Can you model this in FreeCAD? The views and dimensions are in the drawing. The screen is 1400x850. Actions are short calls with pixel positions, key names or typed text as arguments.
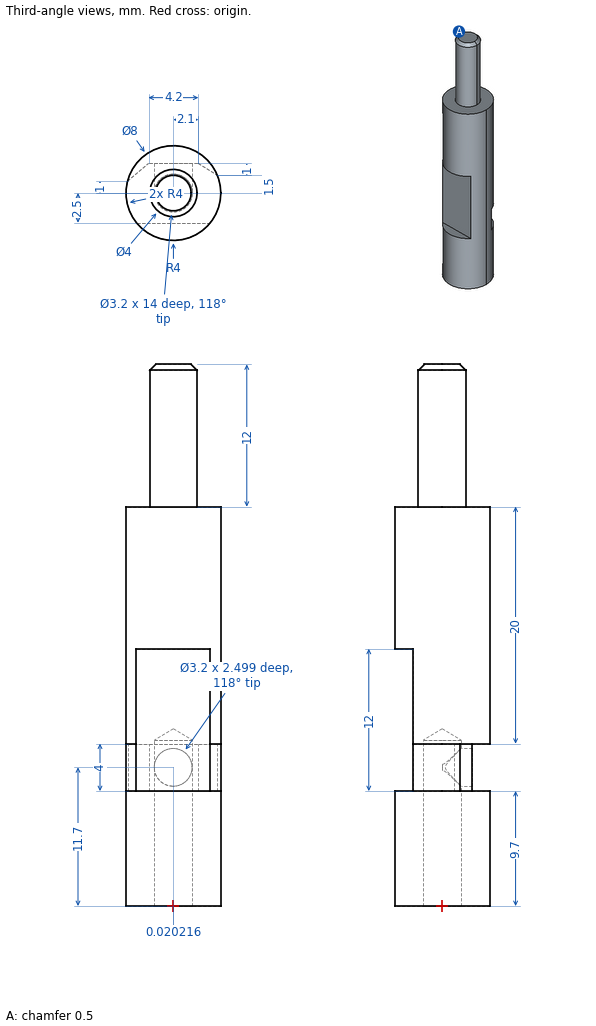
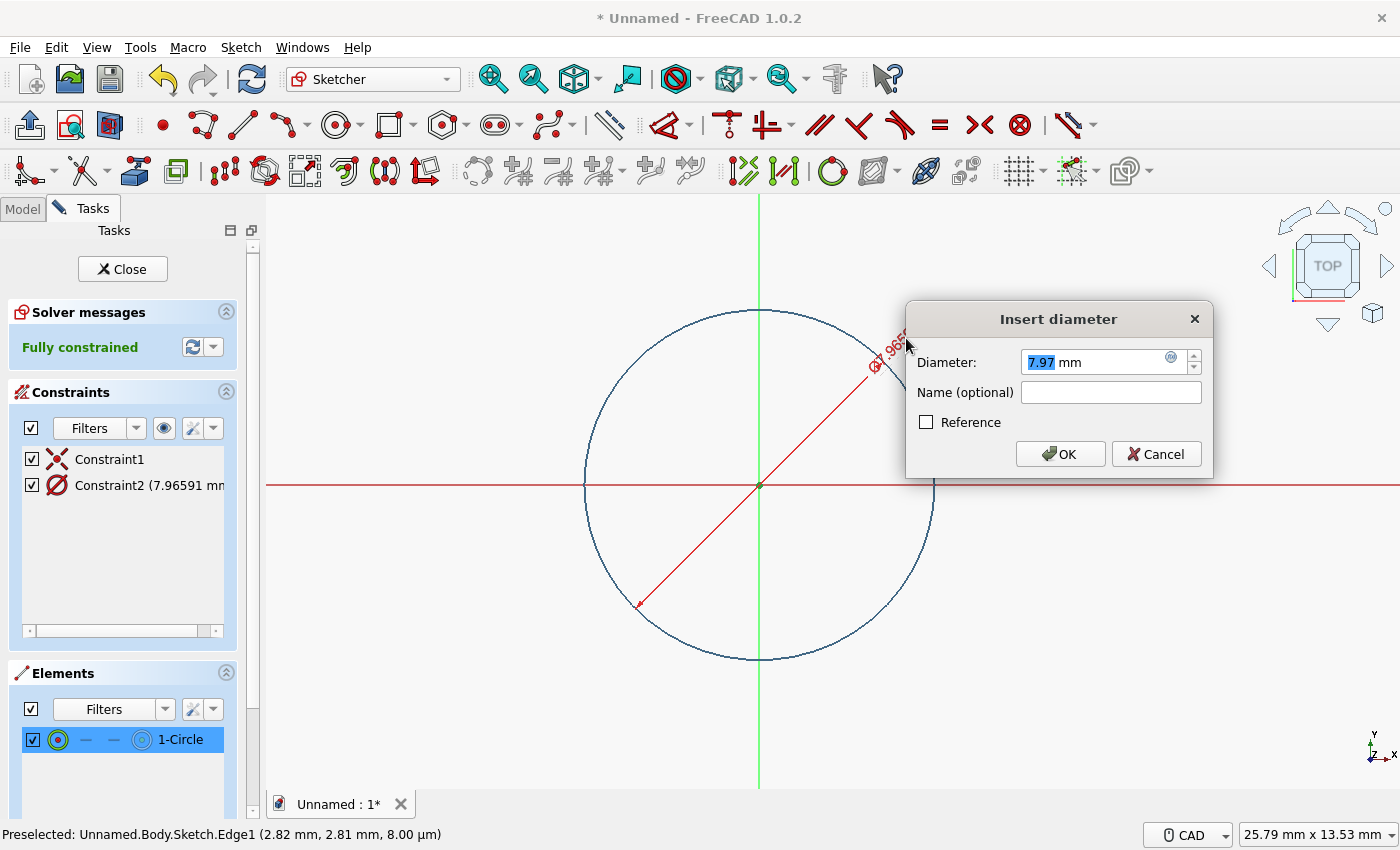
text(8)
key(Return)
key(Escape)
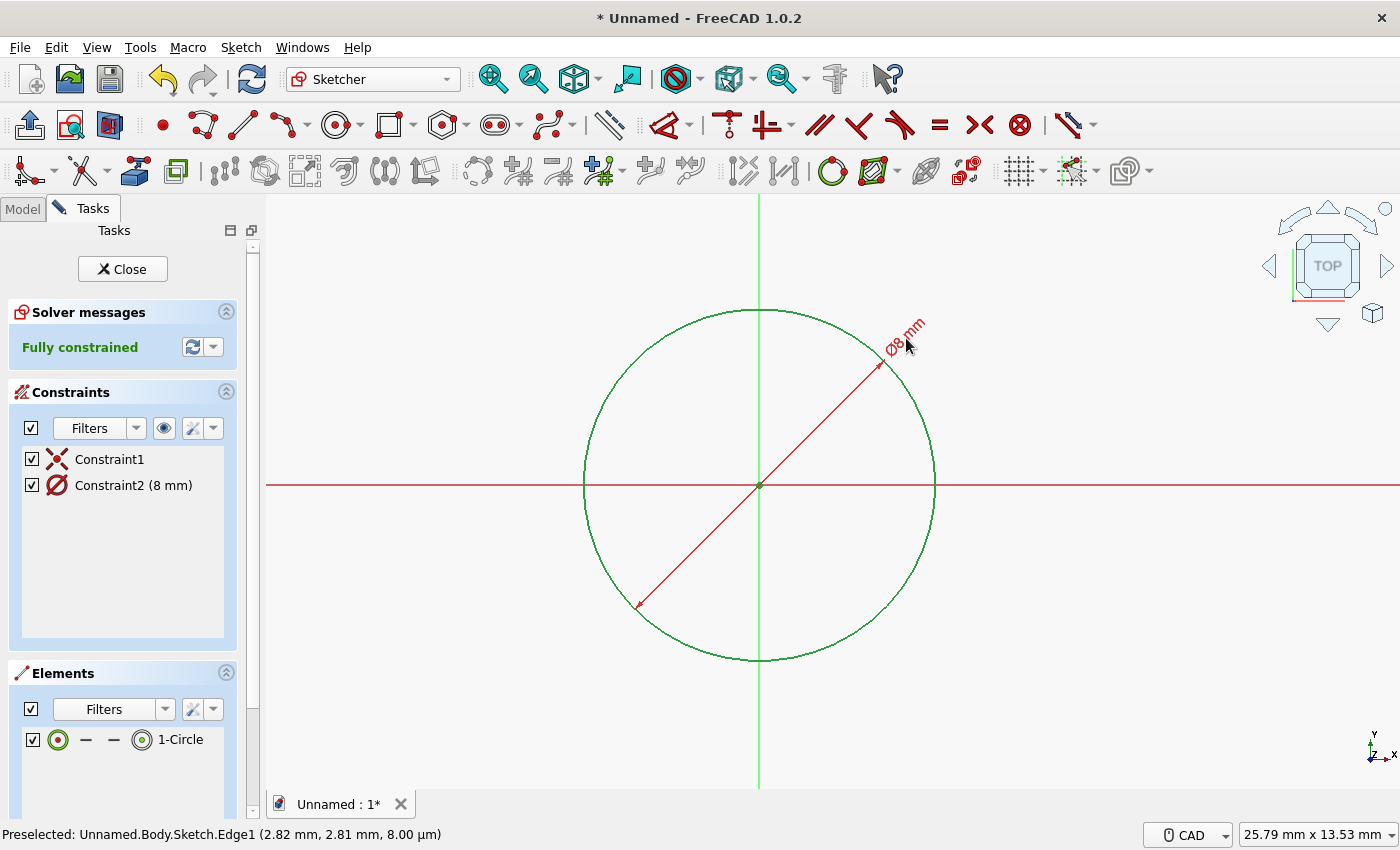
click(123, 269)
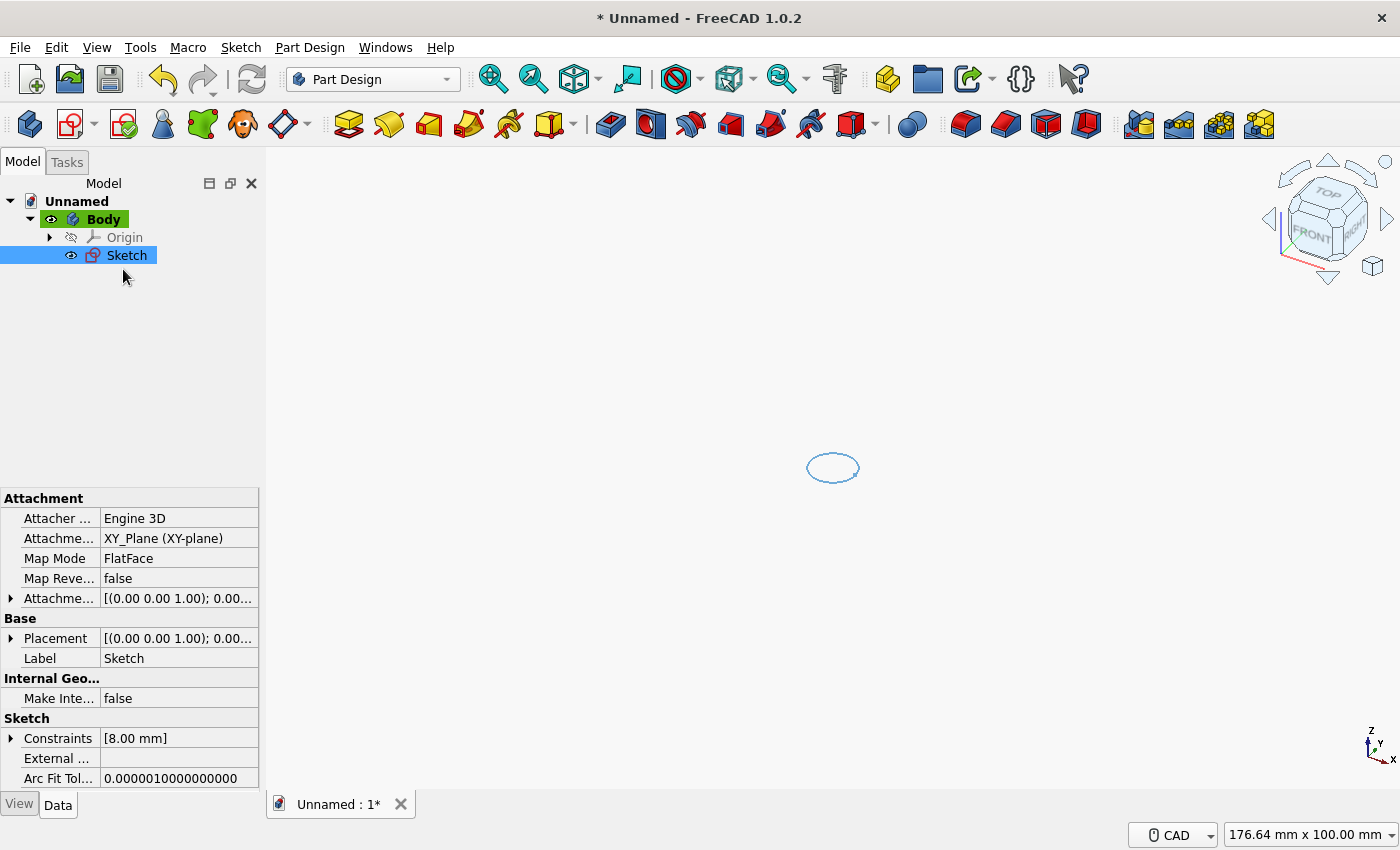
click(350, 124)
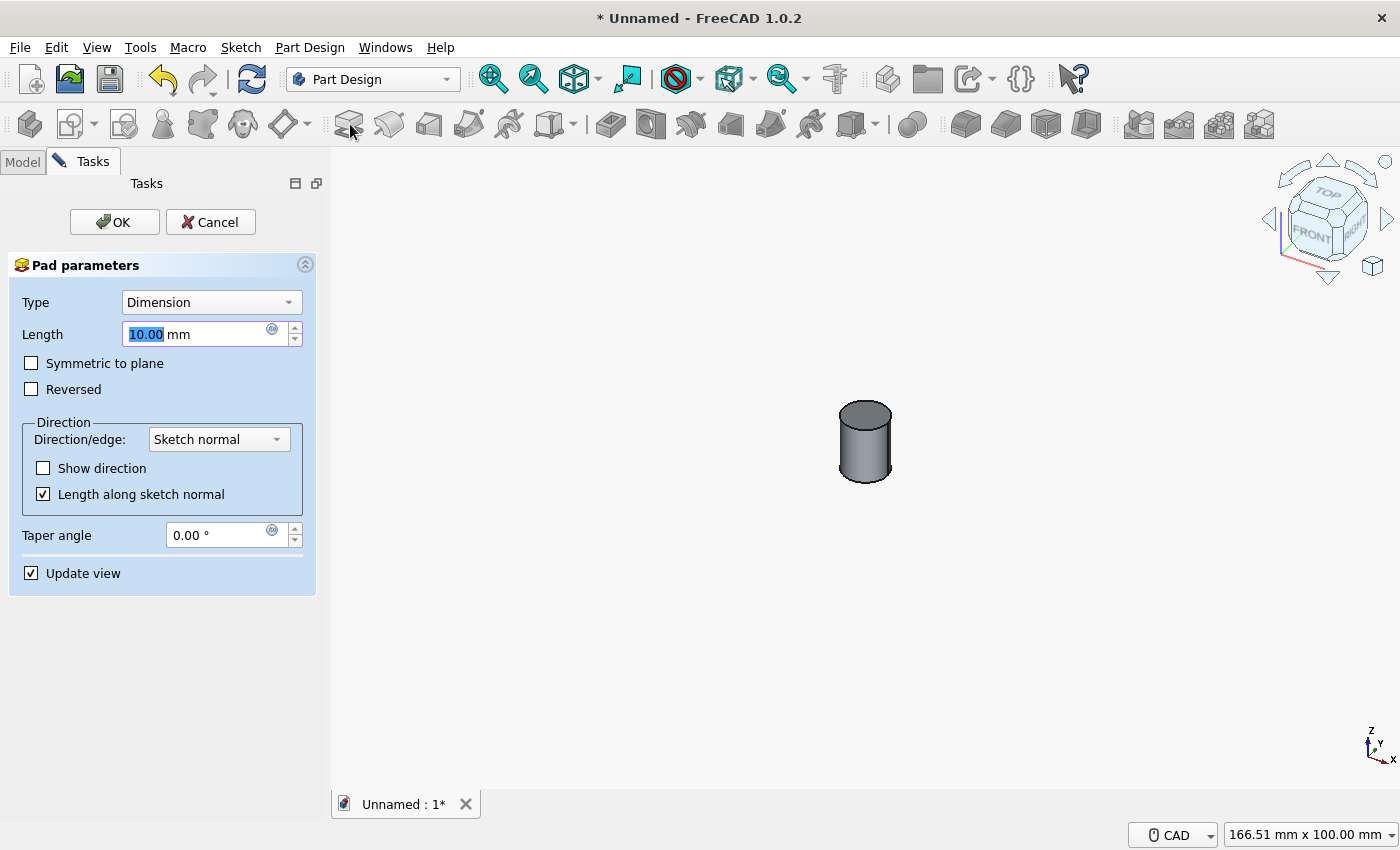
text(9.7)
key(Tab)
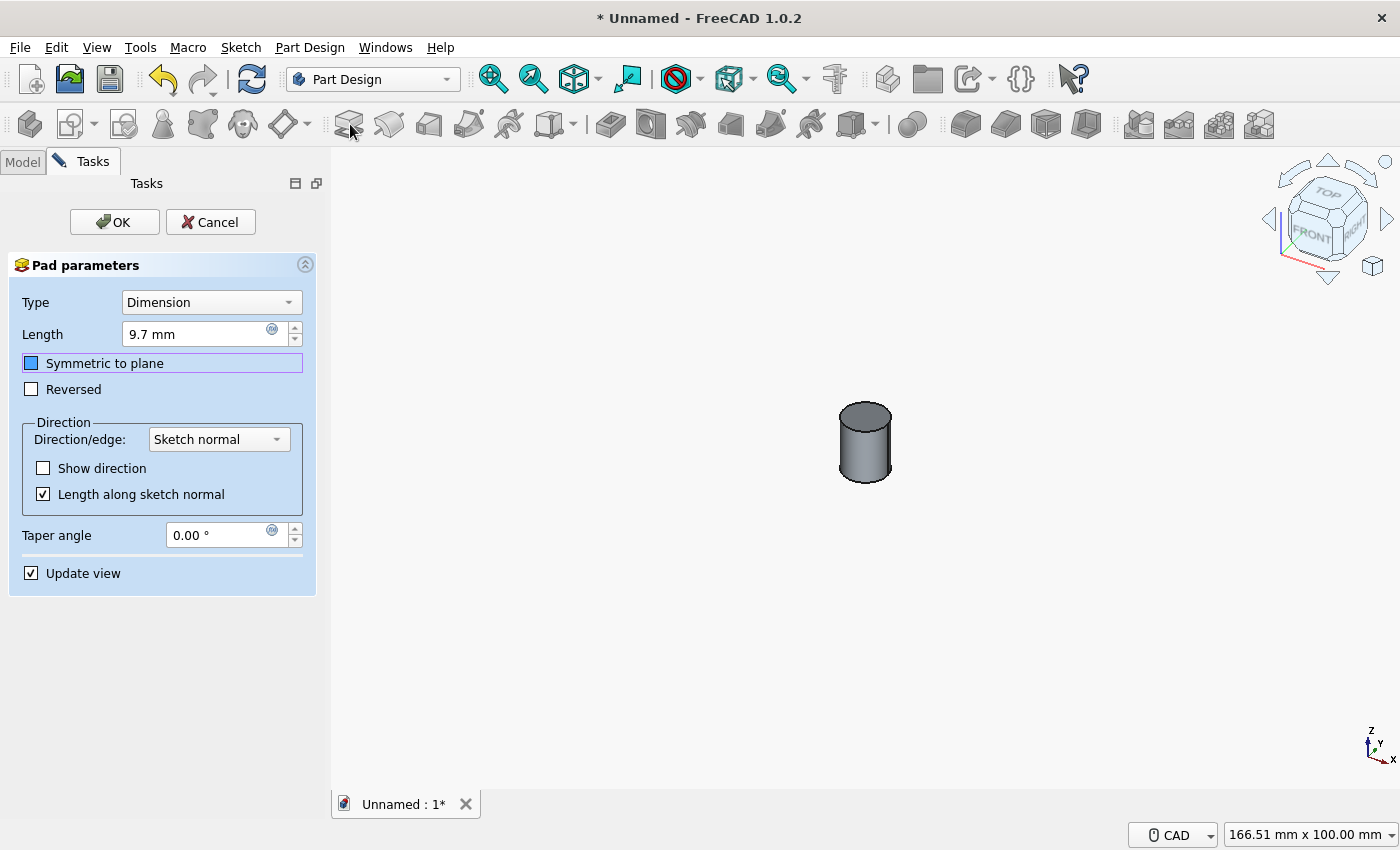
click(115, 222)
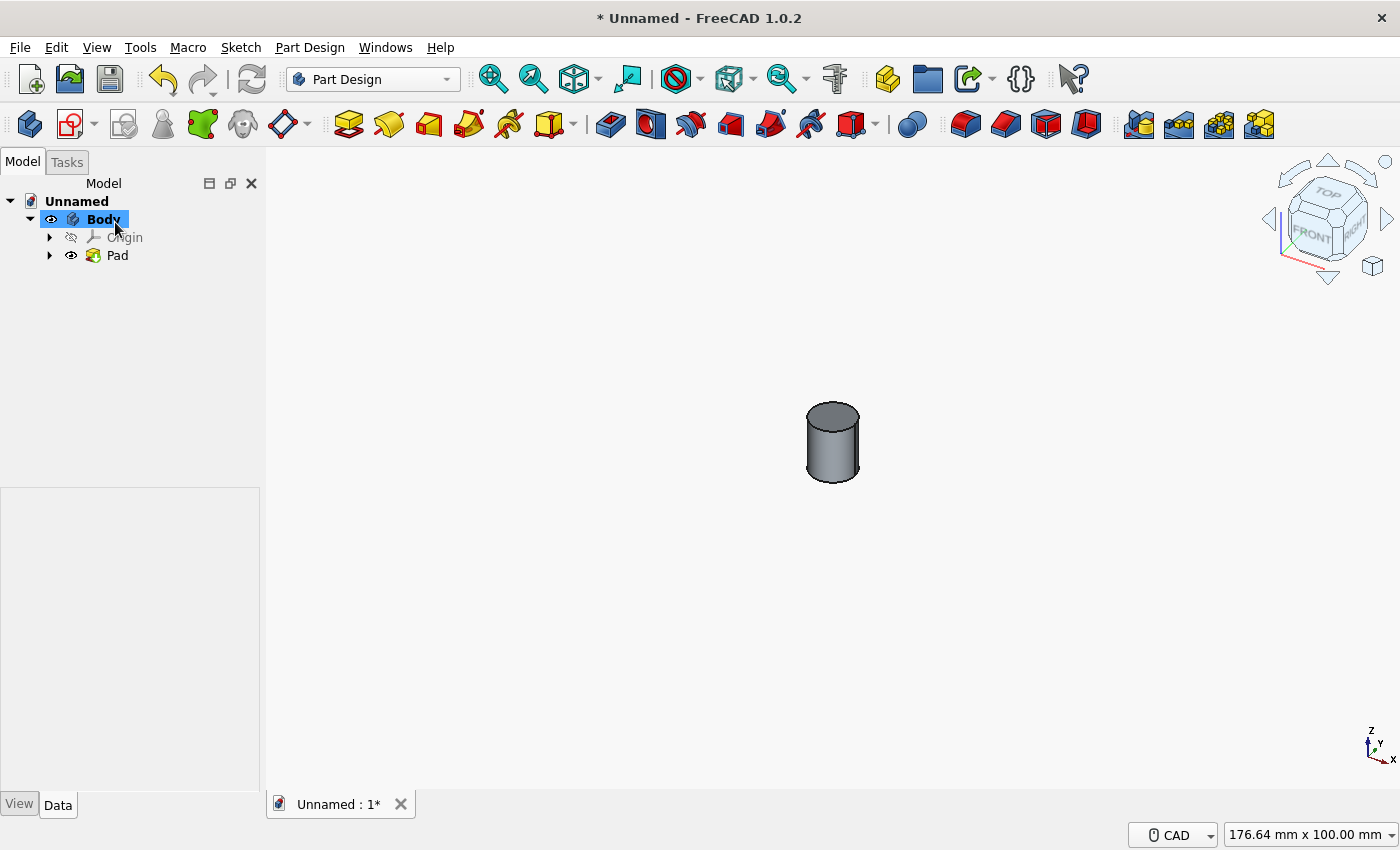
click(494, 80)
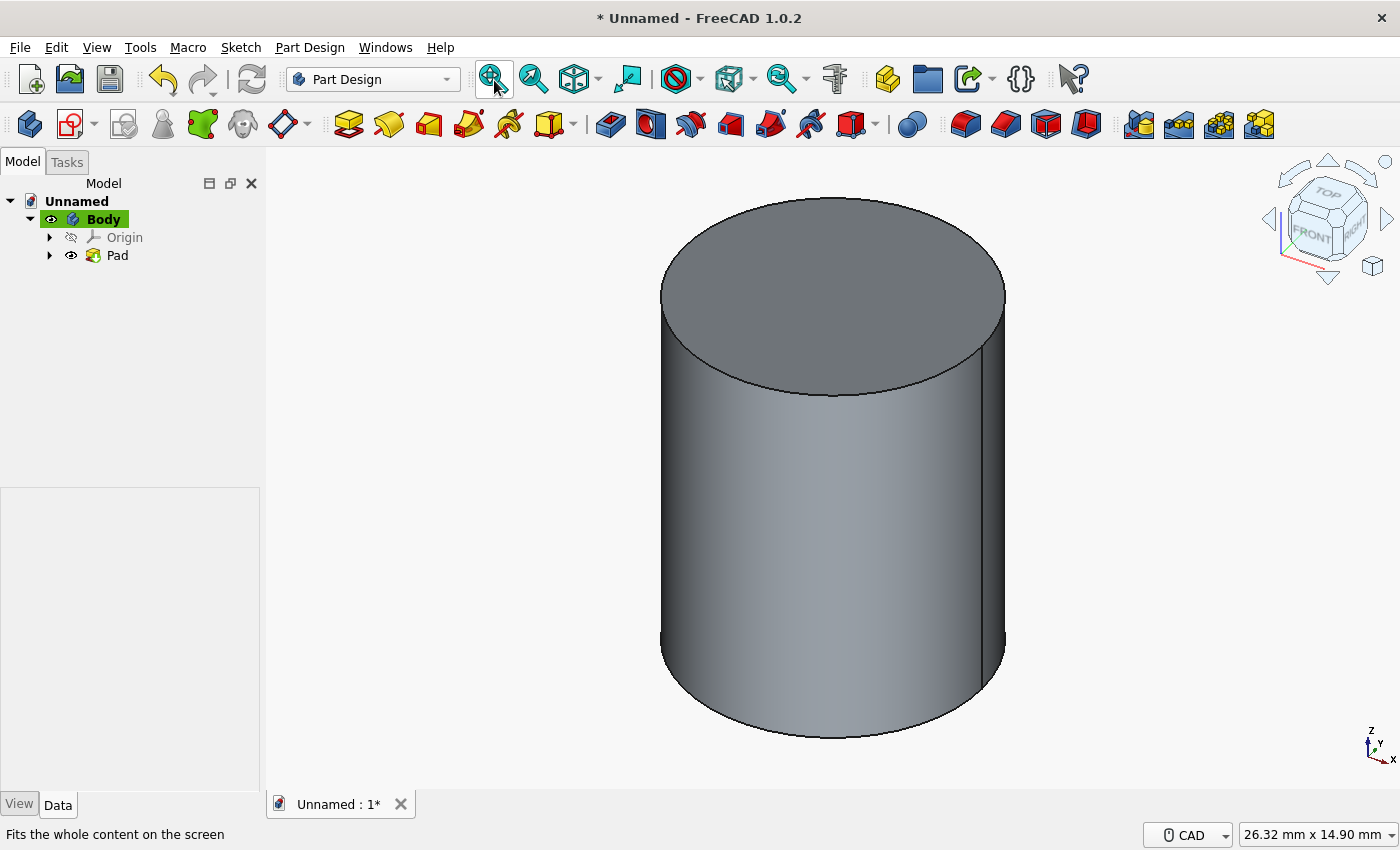
click(833, 296)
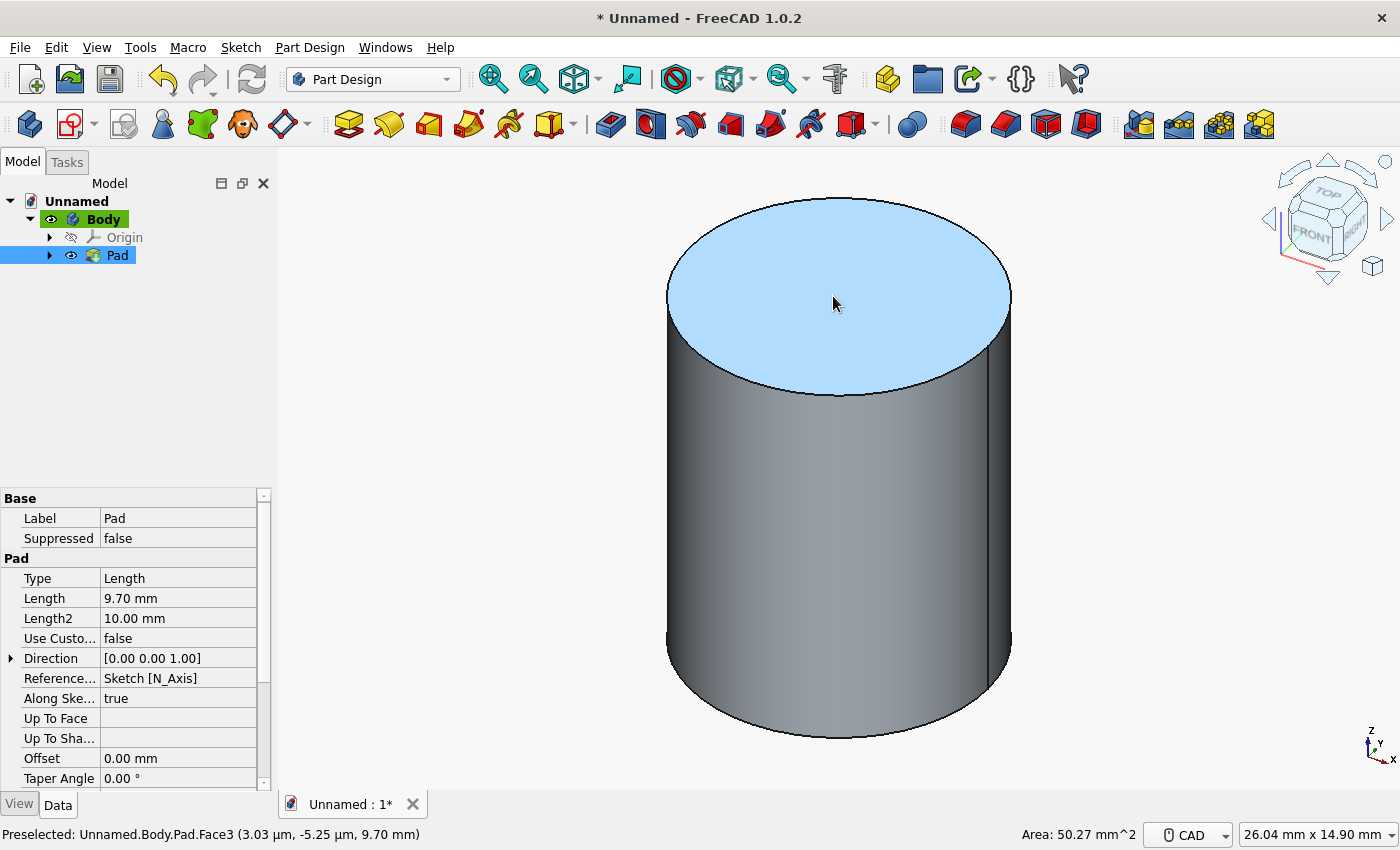
click(70, 124)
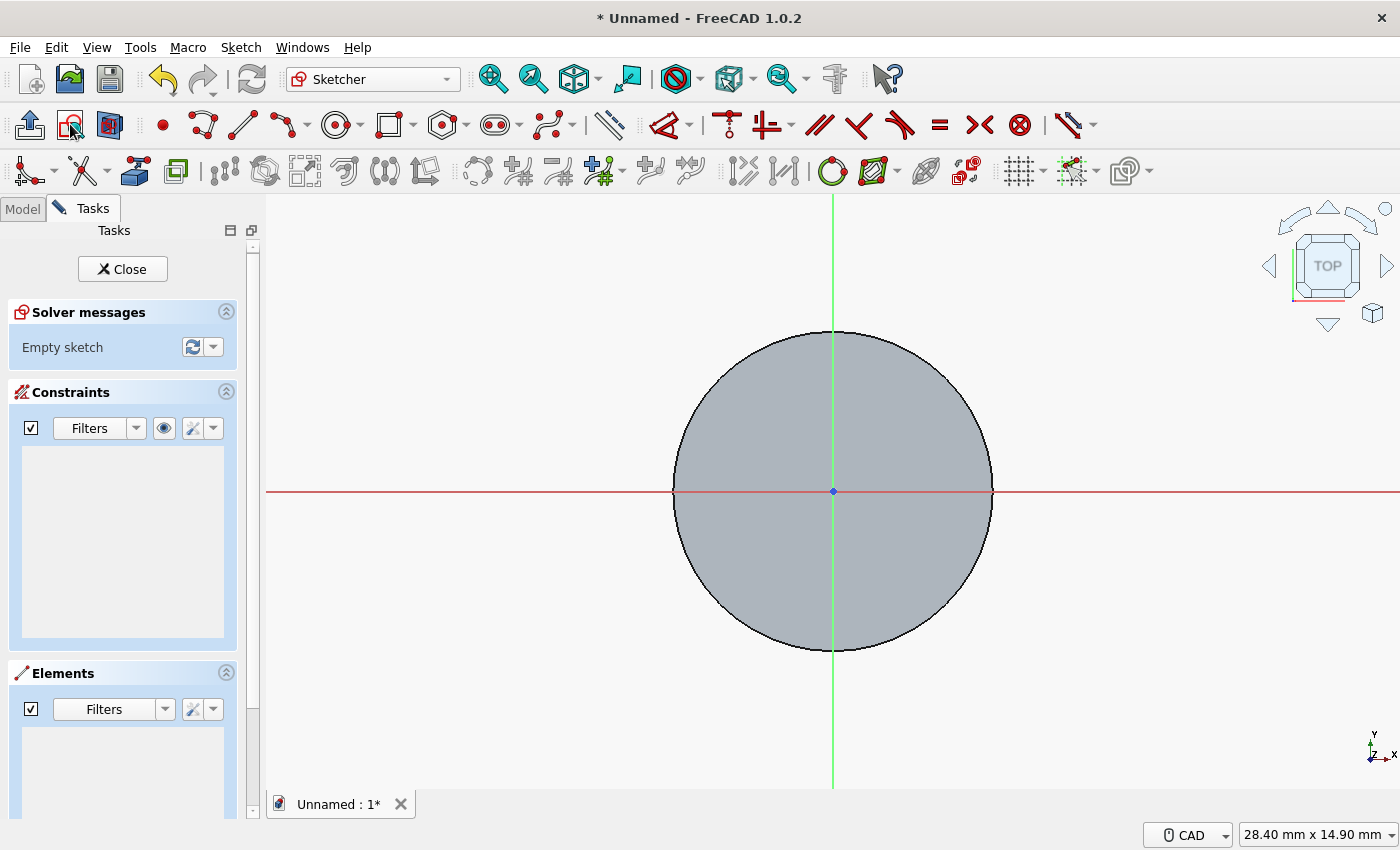
scroll(918, 492, up, 3)